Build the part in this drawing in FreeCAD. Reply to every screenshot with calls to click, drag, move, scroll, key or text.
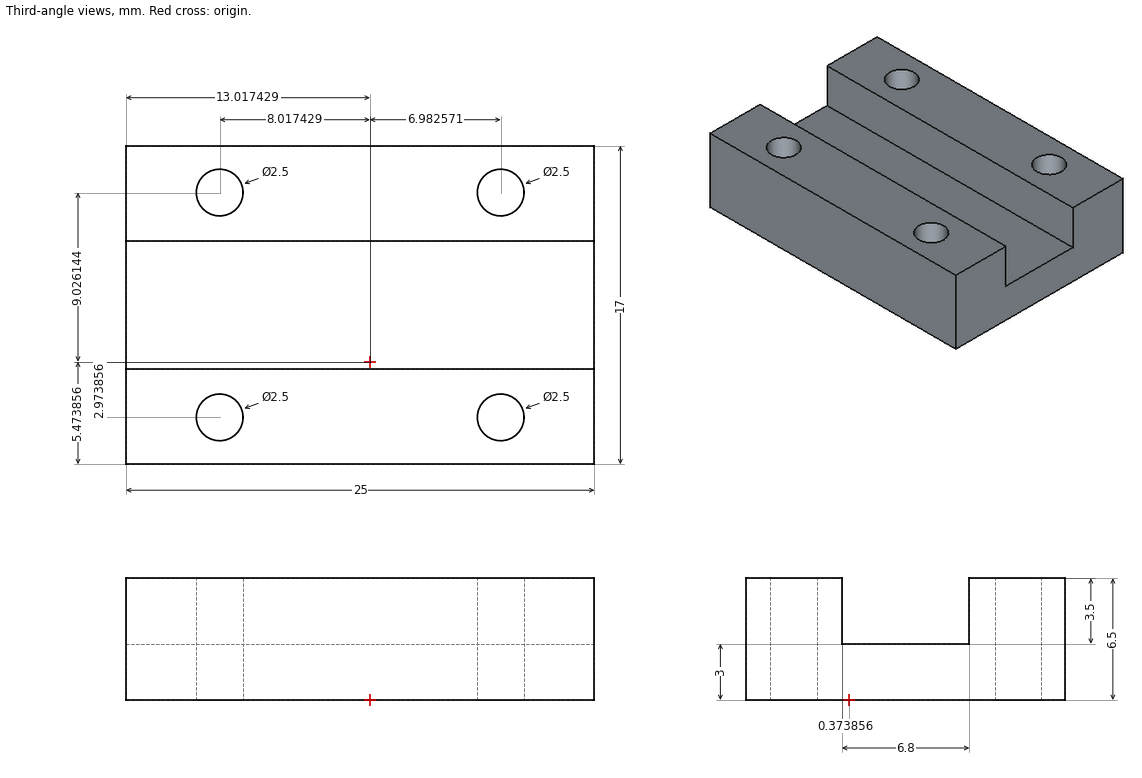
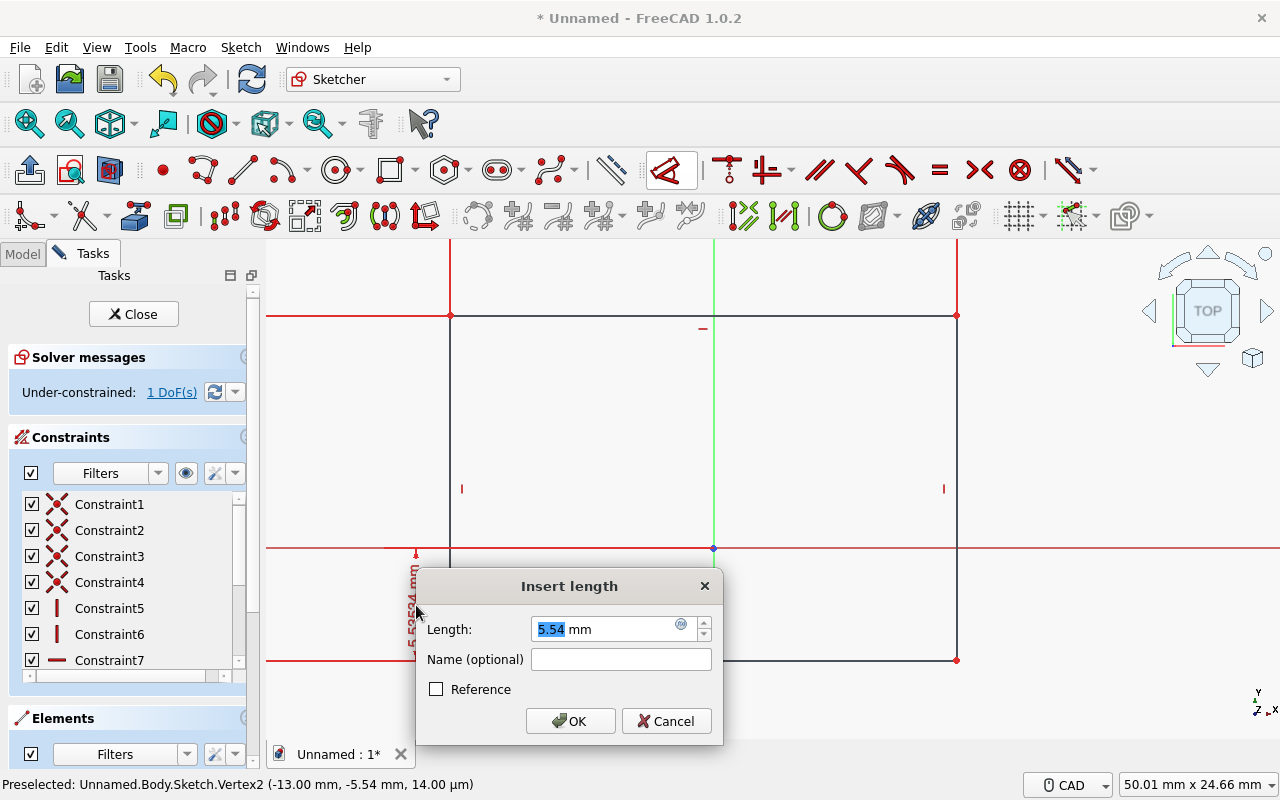
text(5.473856)
key(Return)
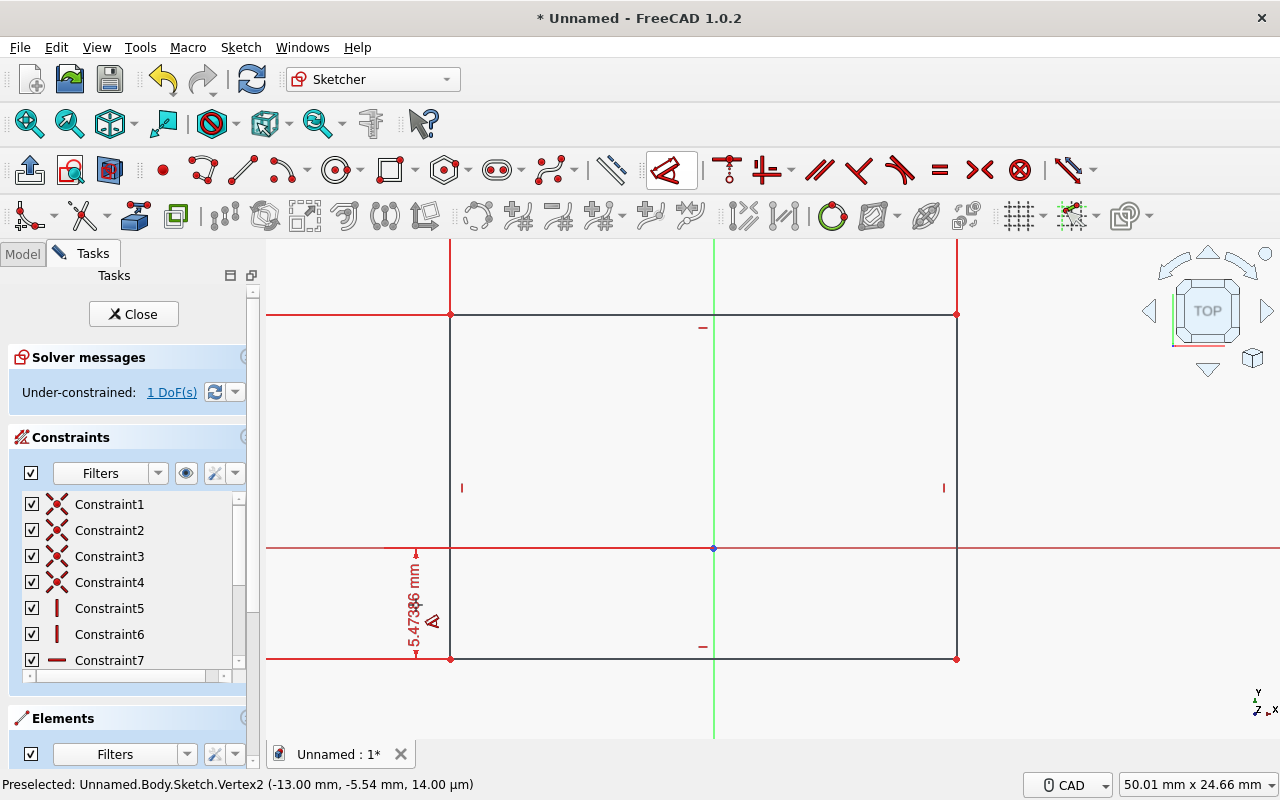
click(450, 315)
click(582, 281)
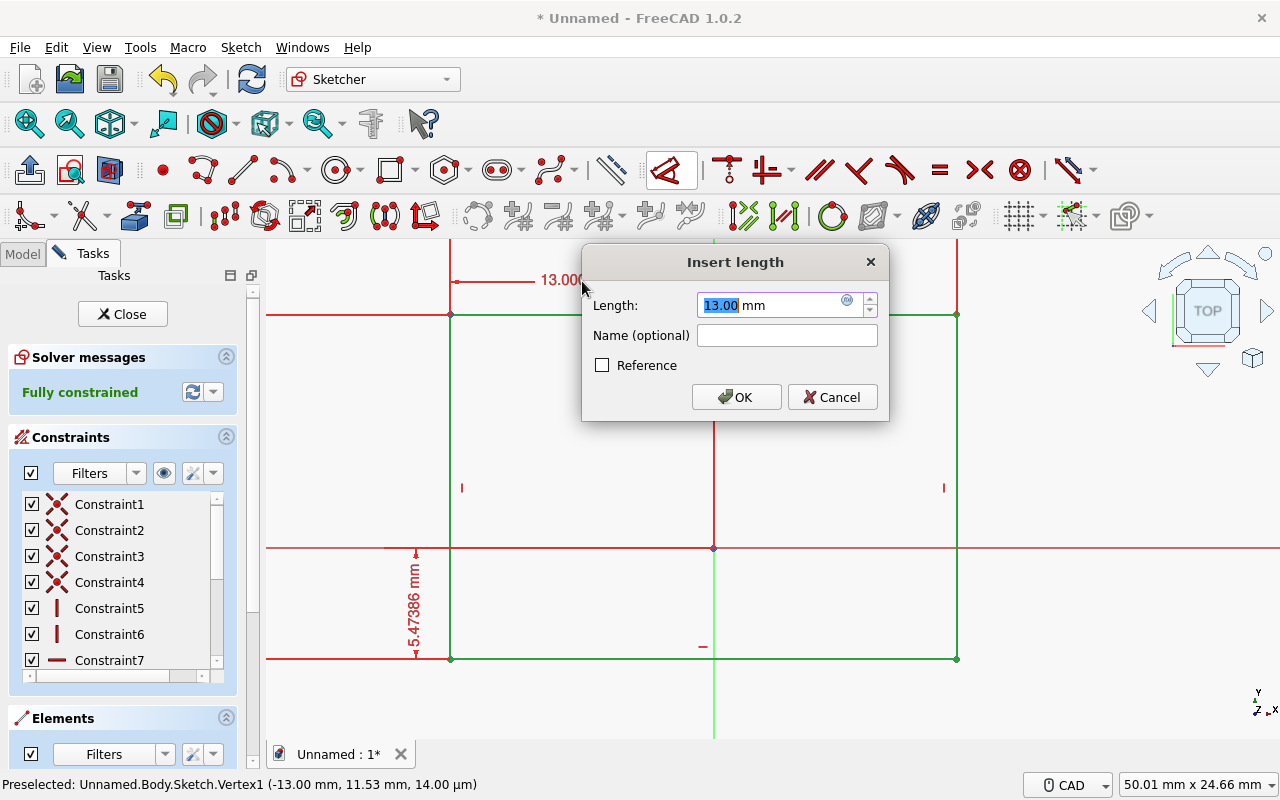
text(13.017429)
key(Return)
key(Escape)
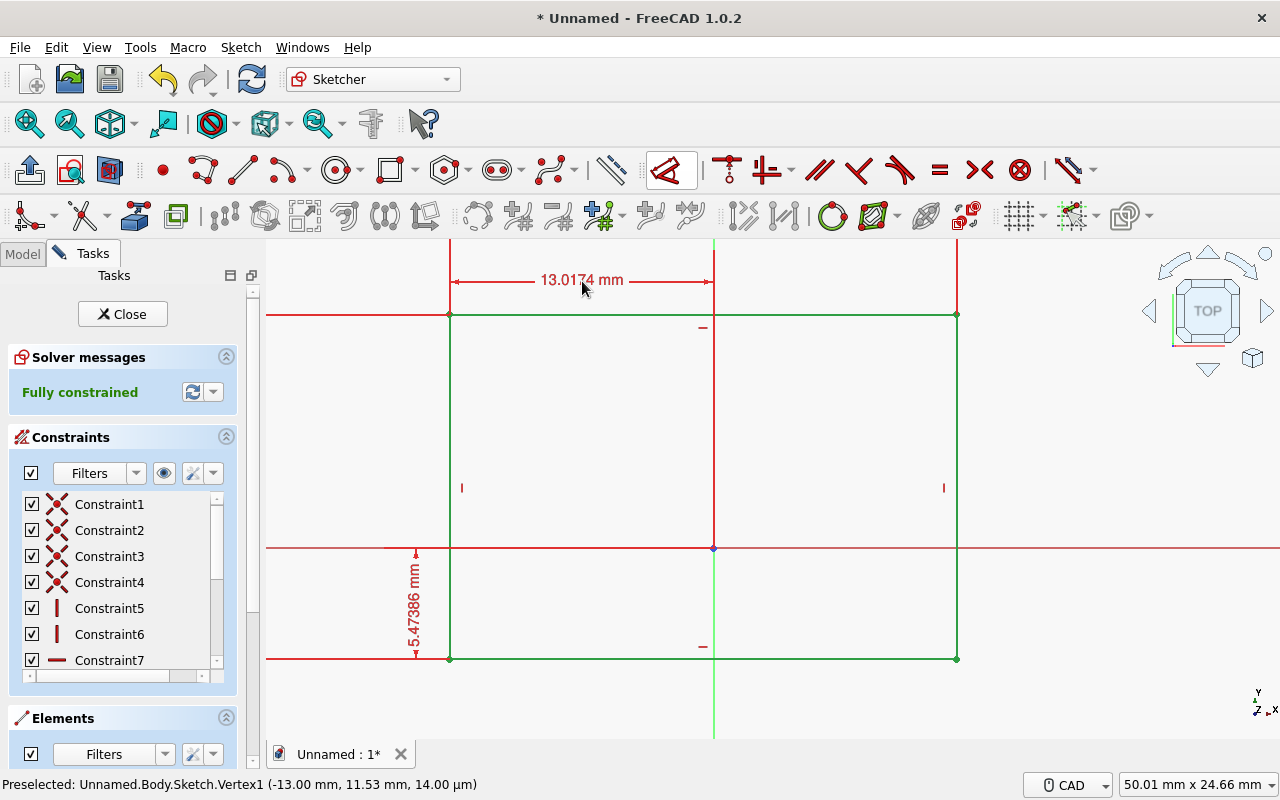
click(123, 314)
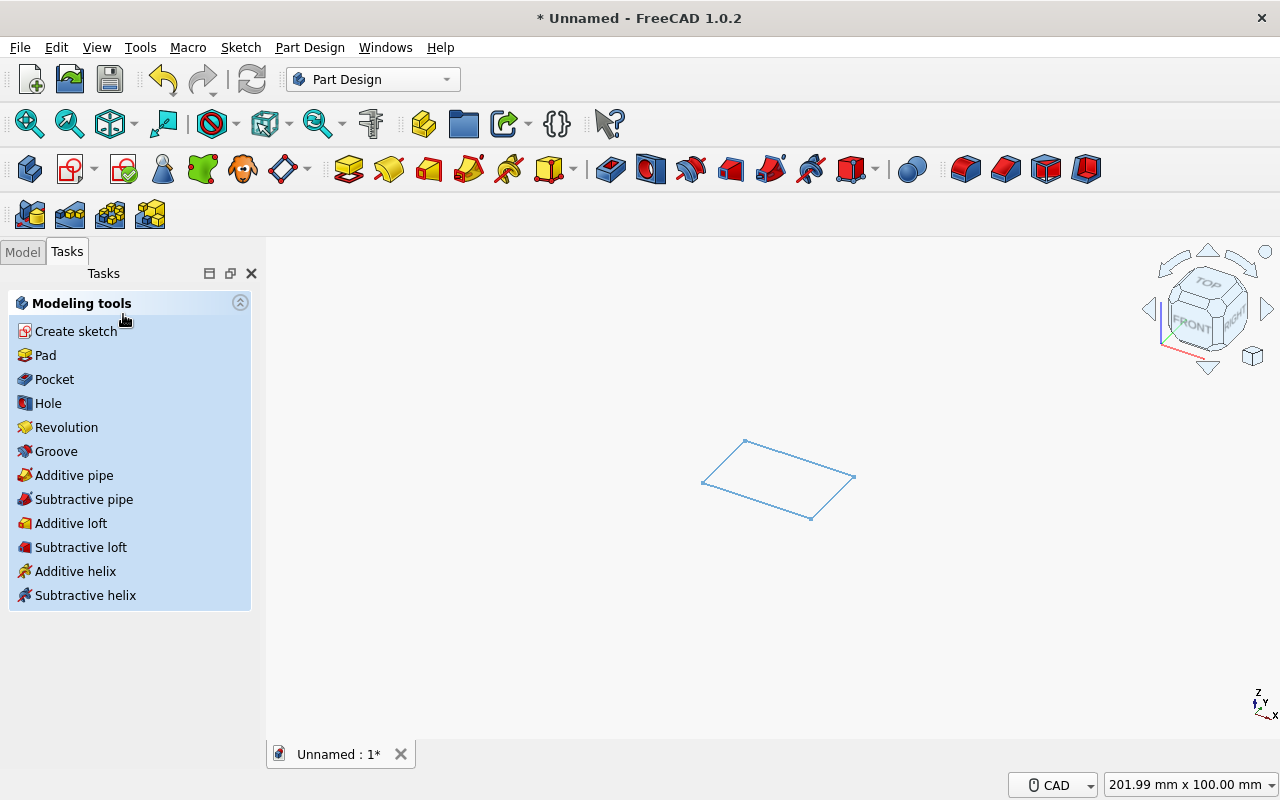
click(350, 170)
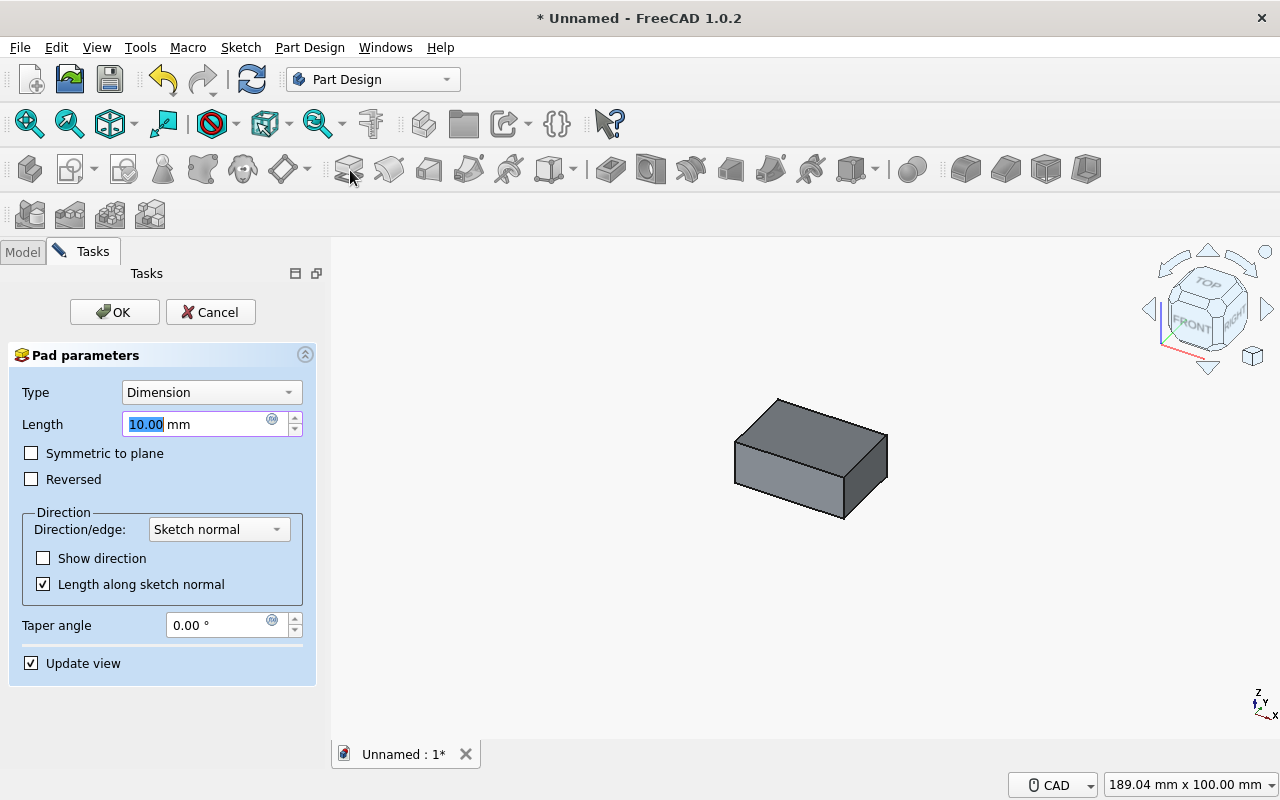
text(6.5)
key(Tab)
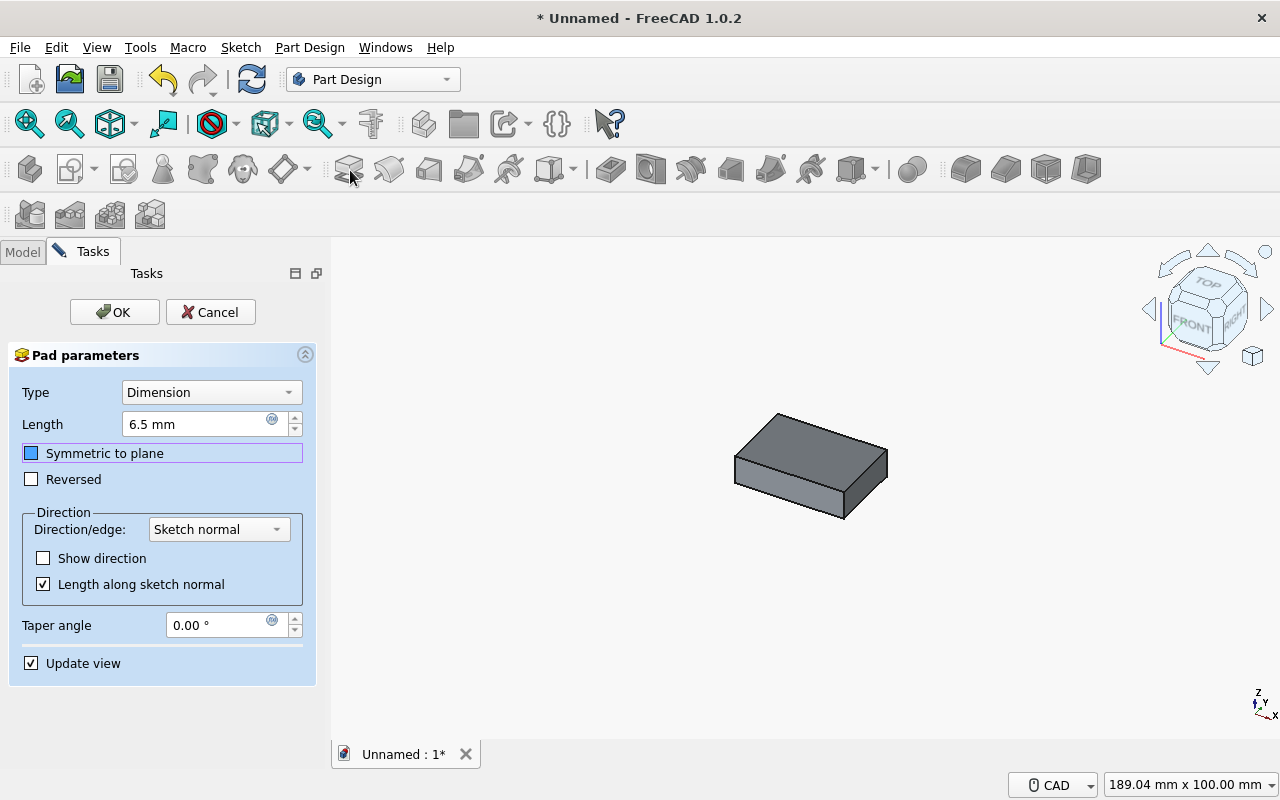
click(115, 312)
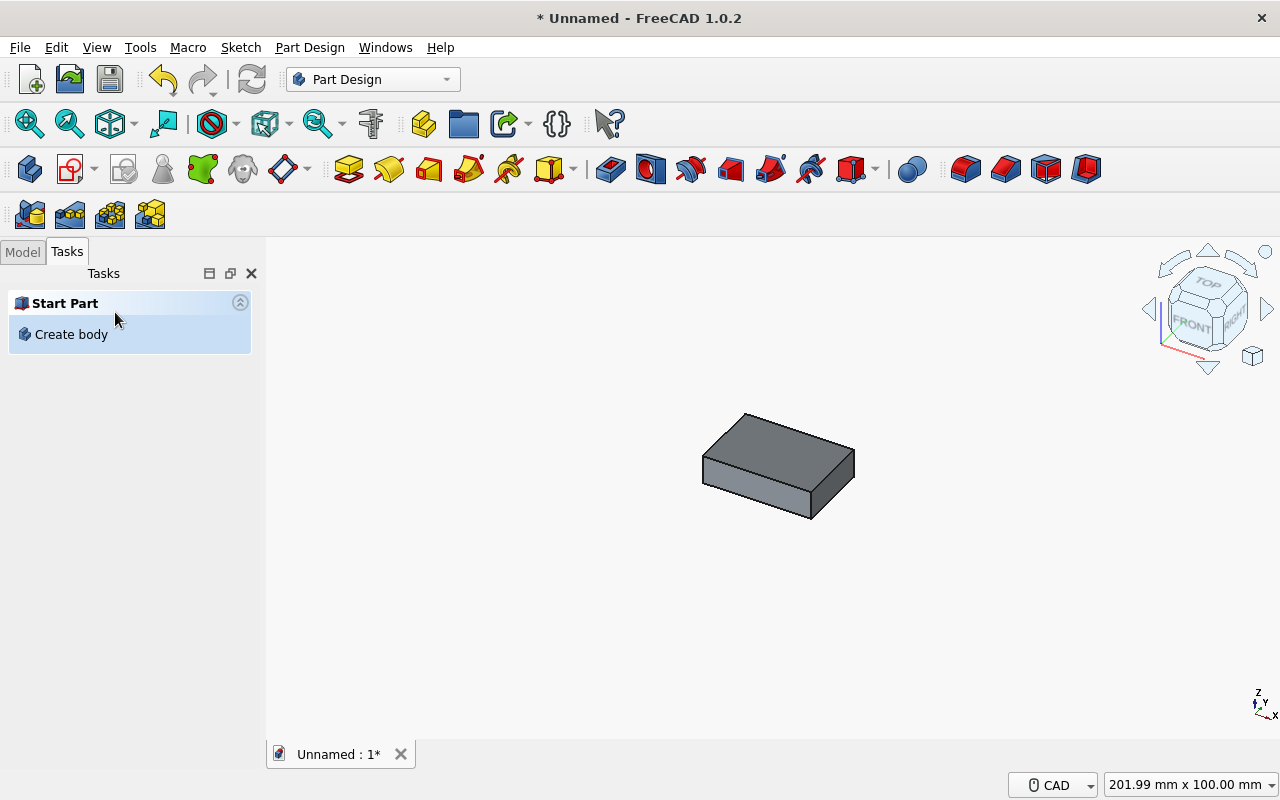
click(30, 124)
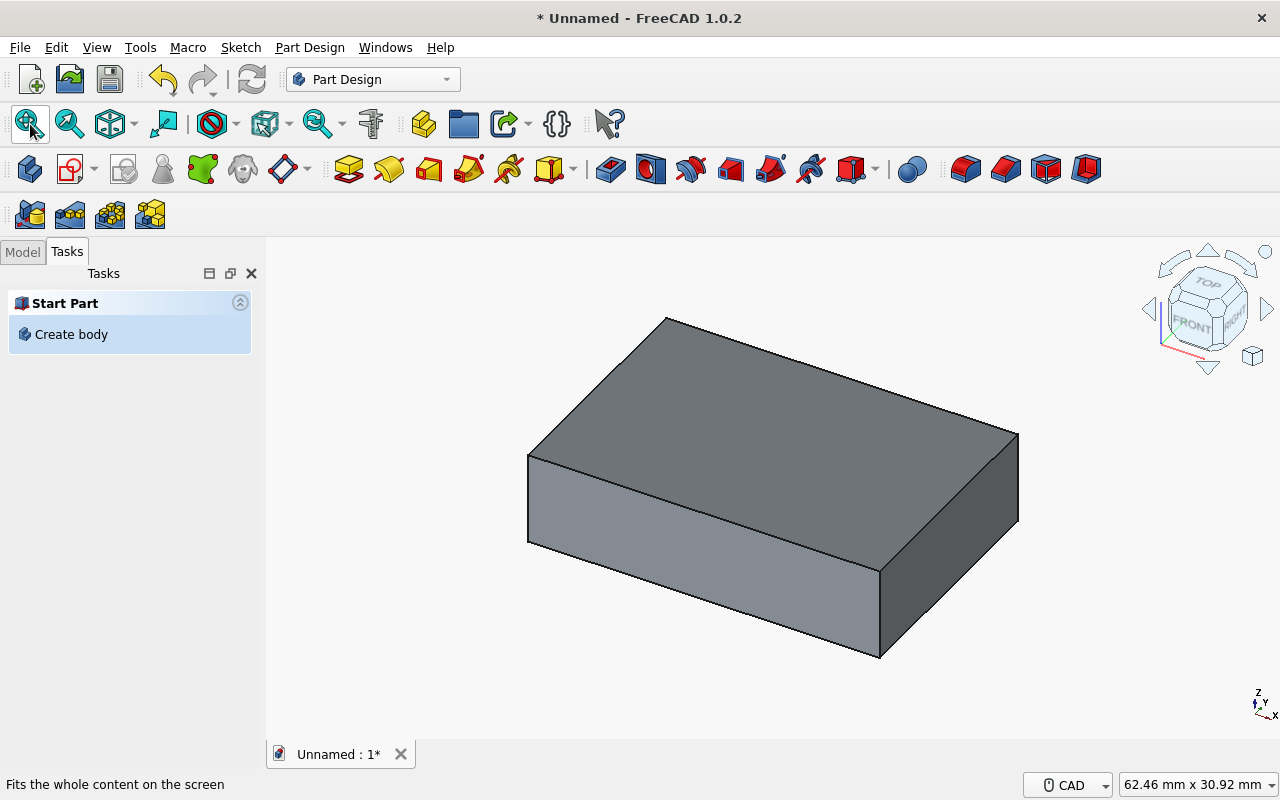
click(988, 506)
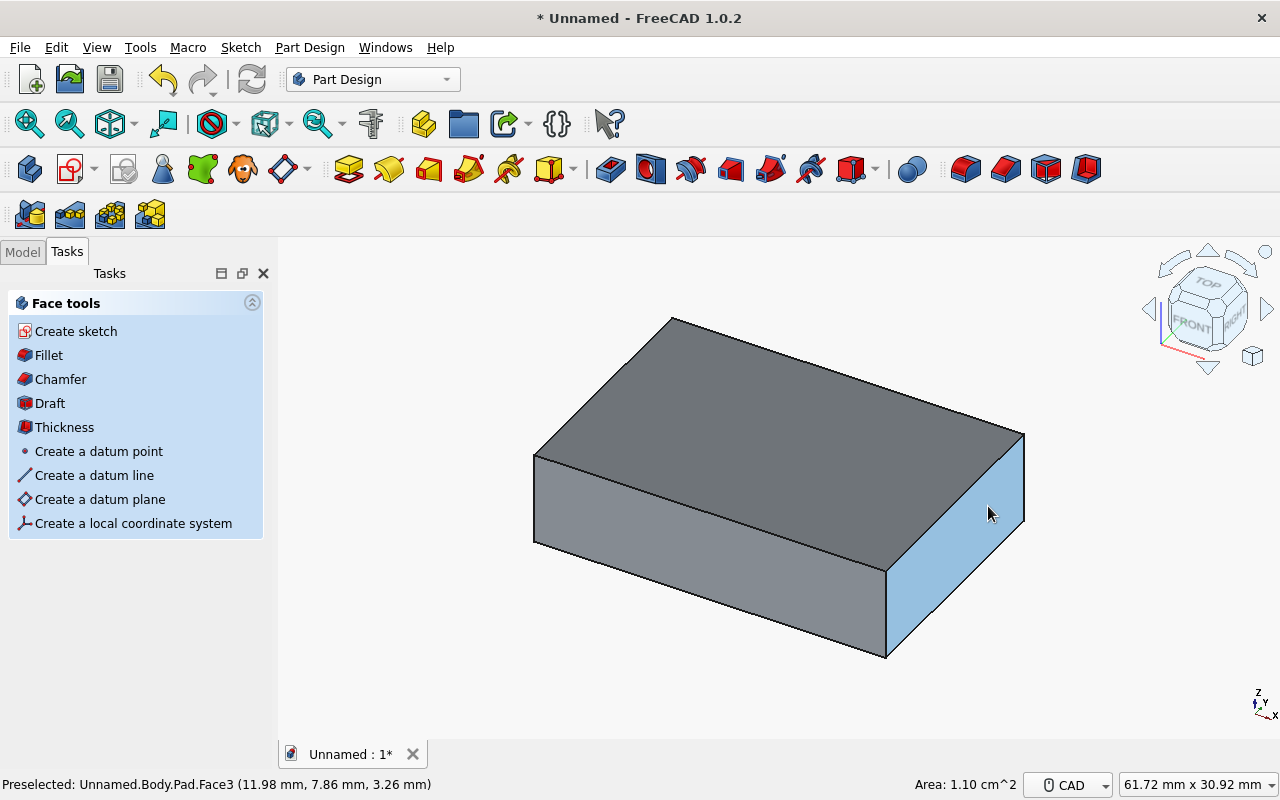
click(70, 170)